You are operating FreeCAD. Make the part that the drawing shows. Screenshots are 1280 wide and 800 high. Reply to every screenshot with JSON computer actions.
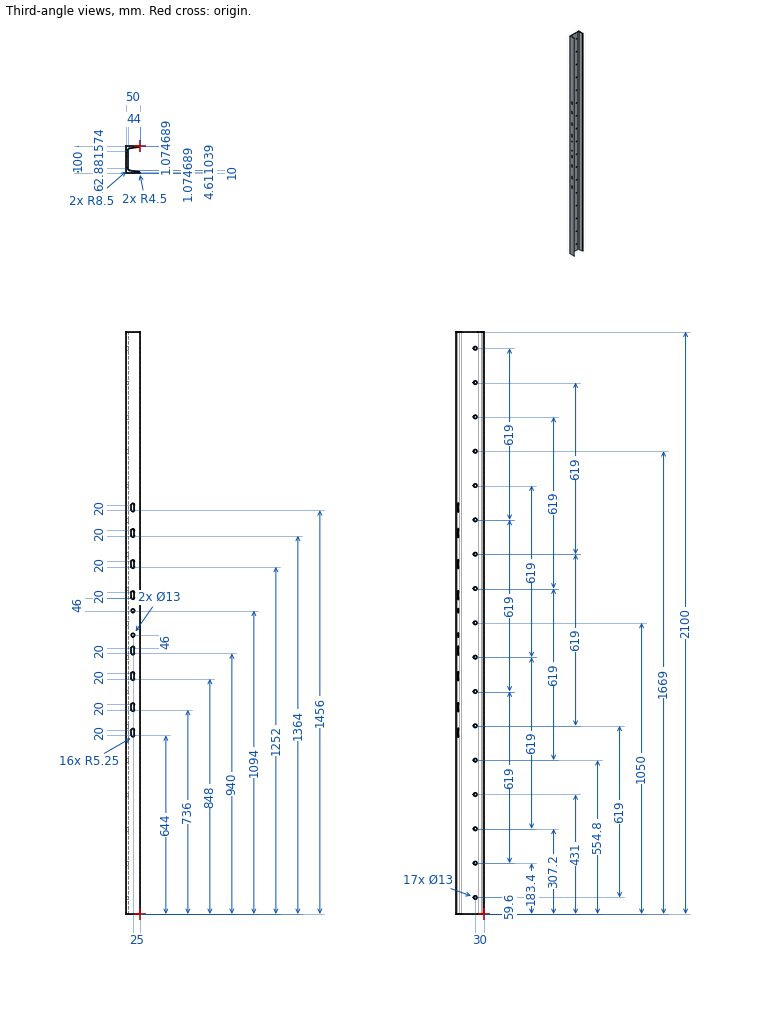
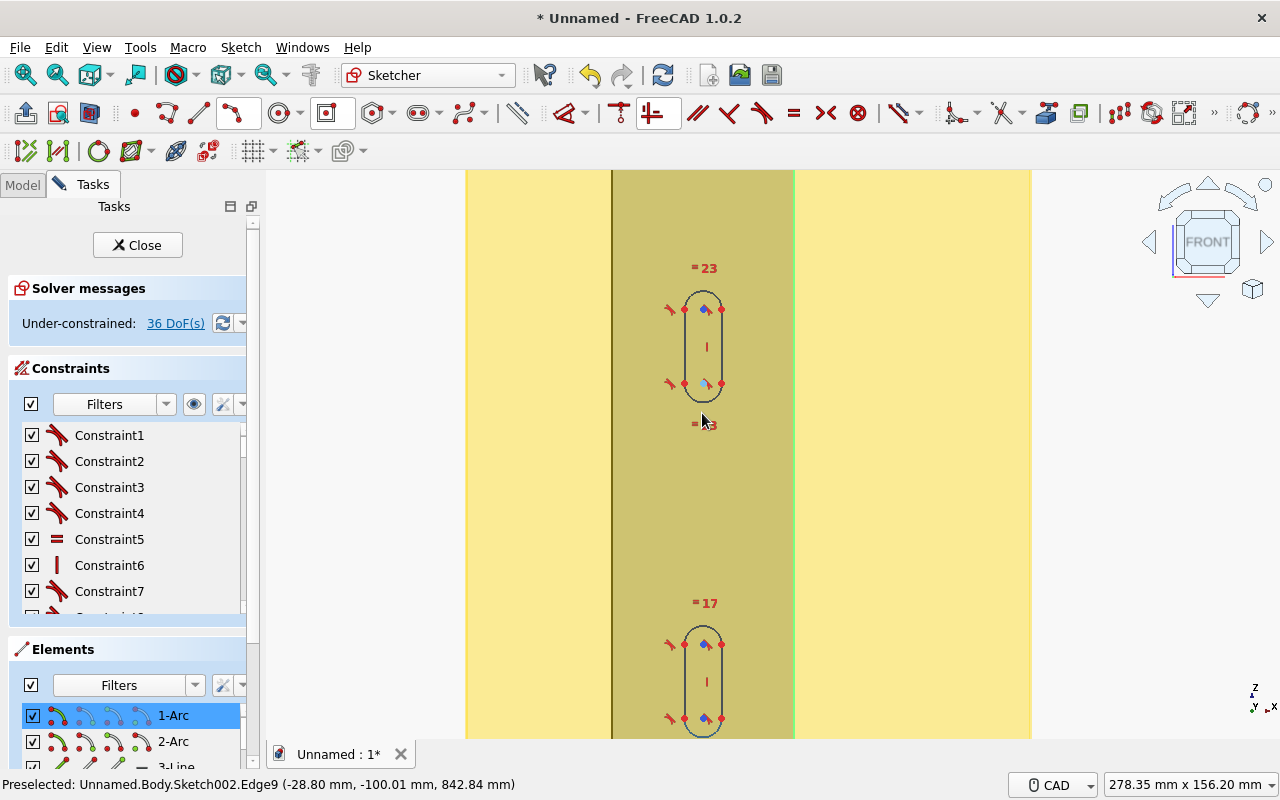
{"action": "left_click", "coordinate": [693, 399]}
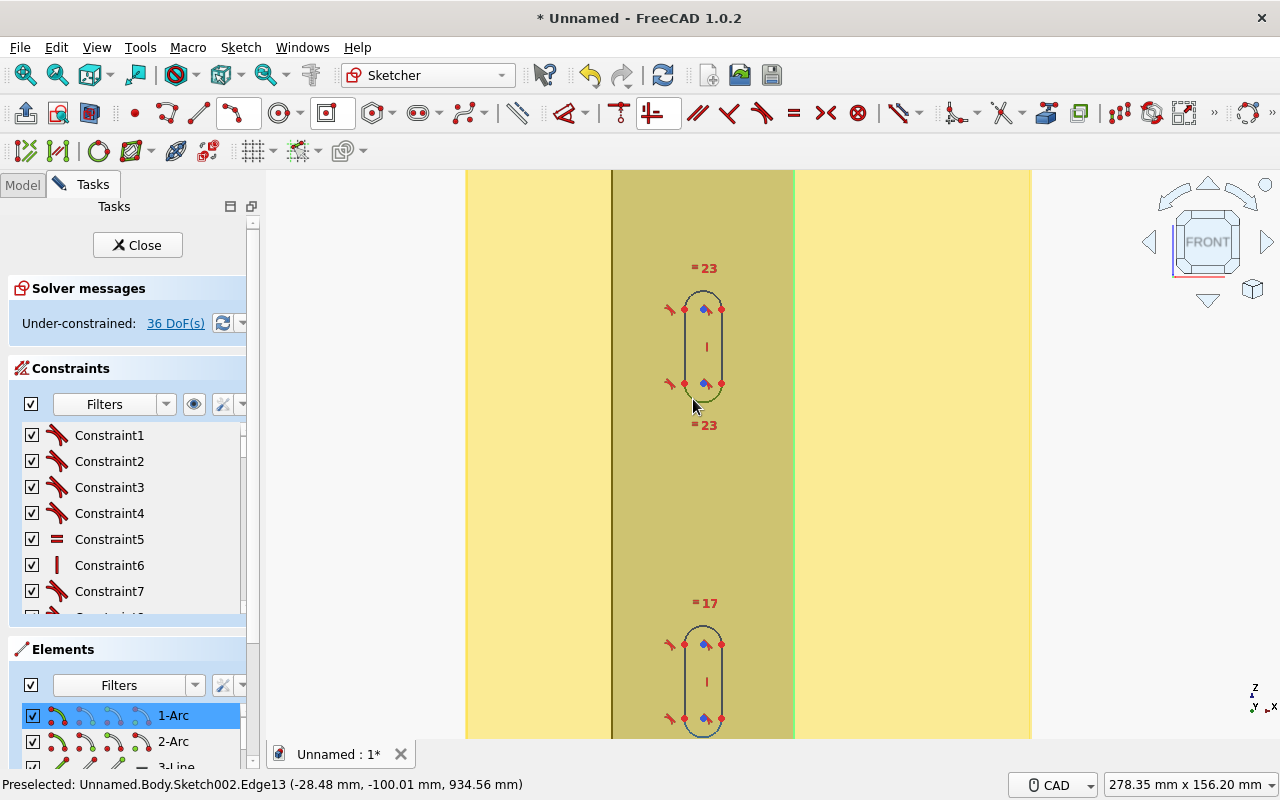
{"action": "scroll", "coordinate": [702, 413], "scroll_direction": "down", "scroll_amount": 14}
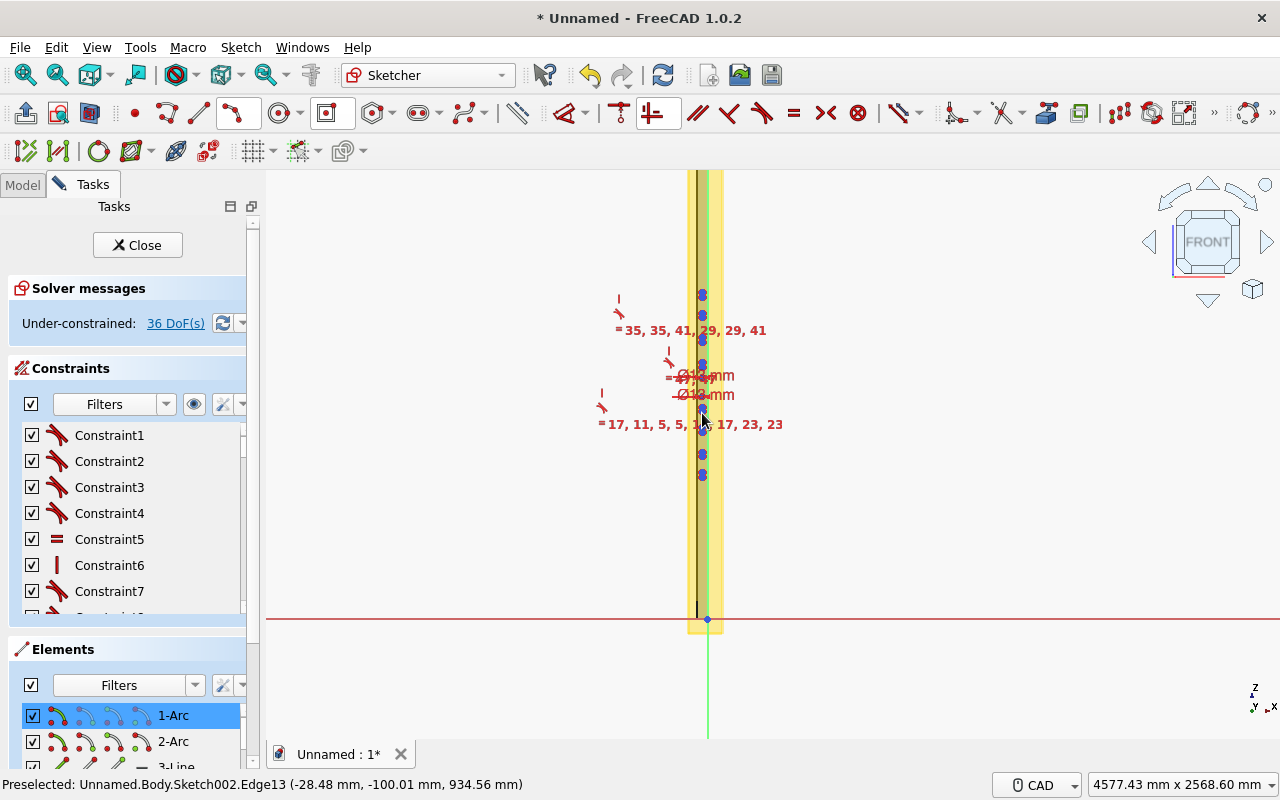
{"action": "scroll", "coordinate": [702, 343], "scroll_direction": "up", "scroll_amount": 14}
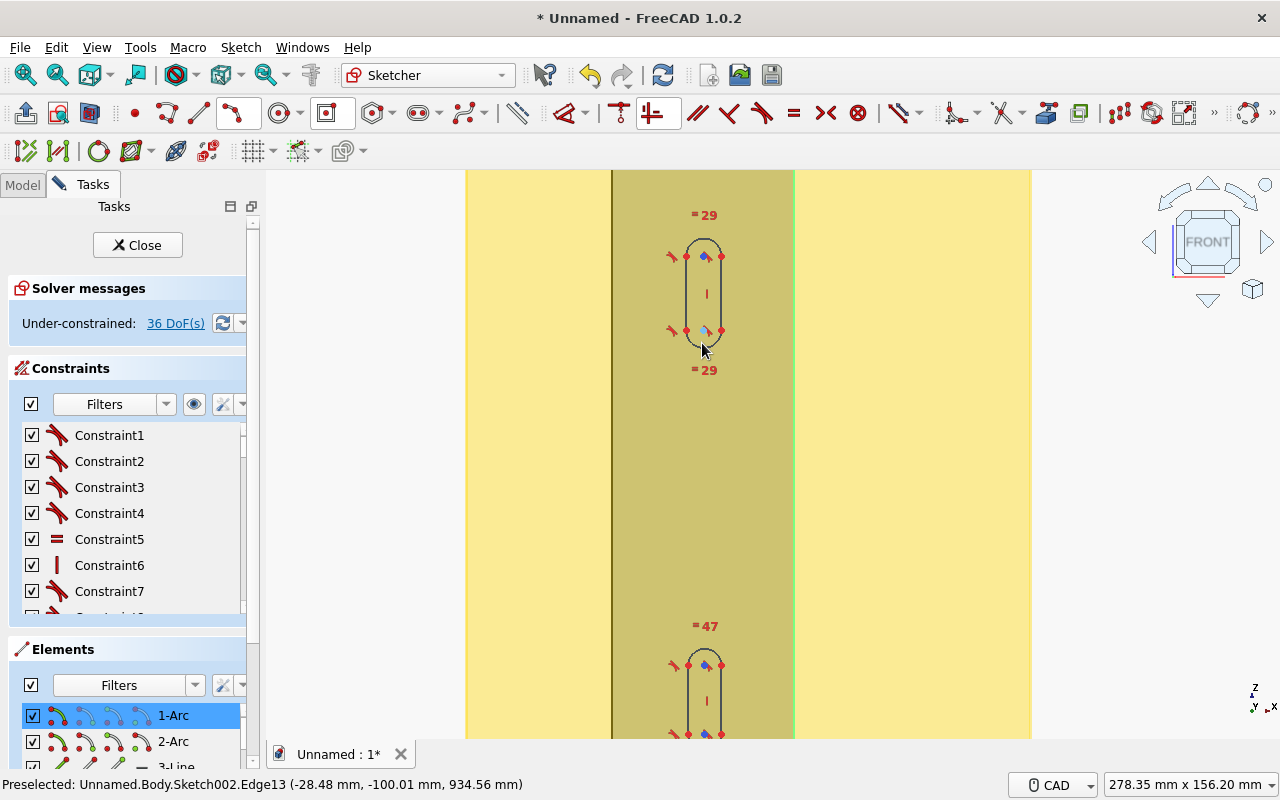
{"action": "left_click", "coordinate": [693, 345]}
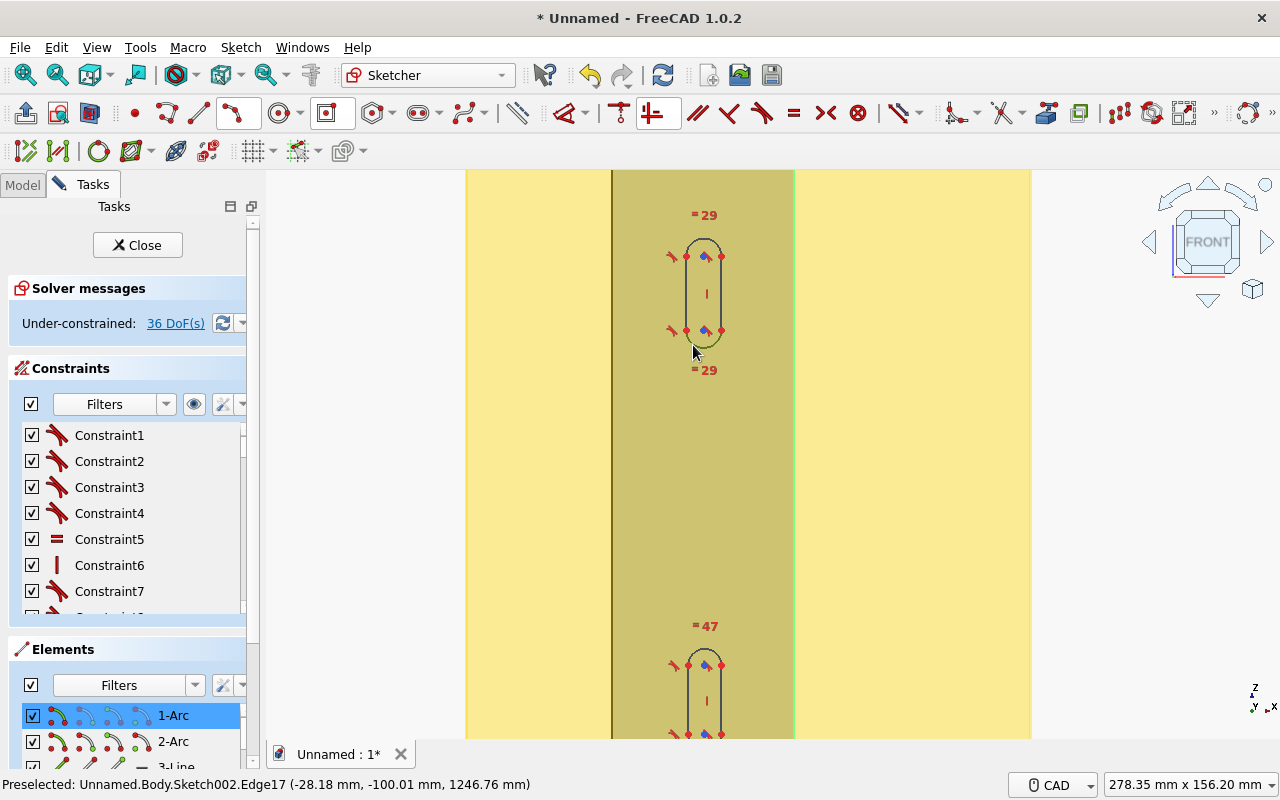
{"action": "scroll", "coordinate": [702, 342], "scroll_direction": "down", "scroll_amount": 14}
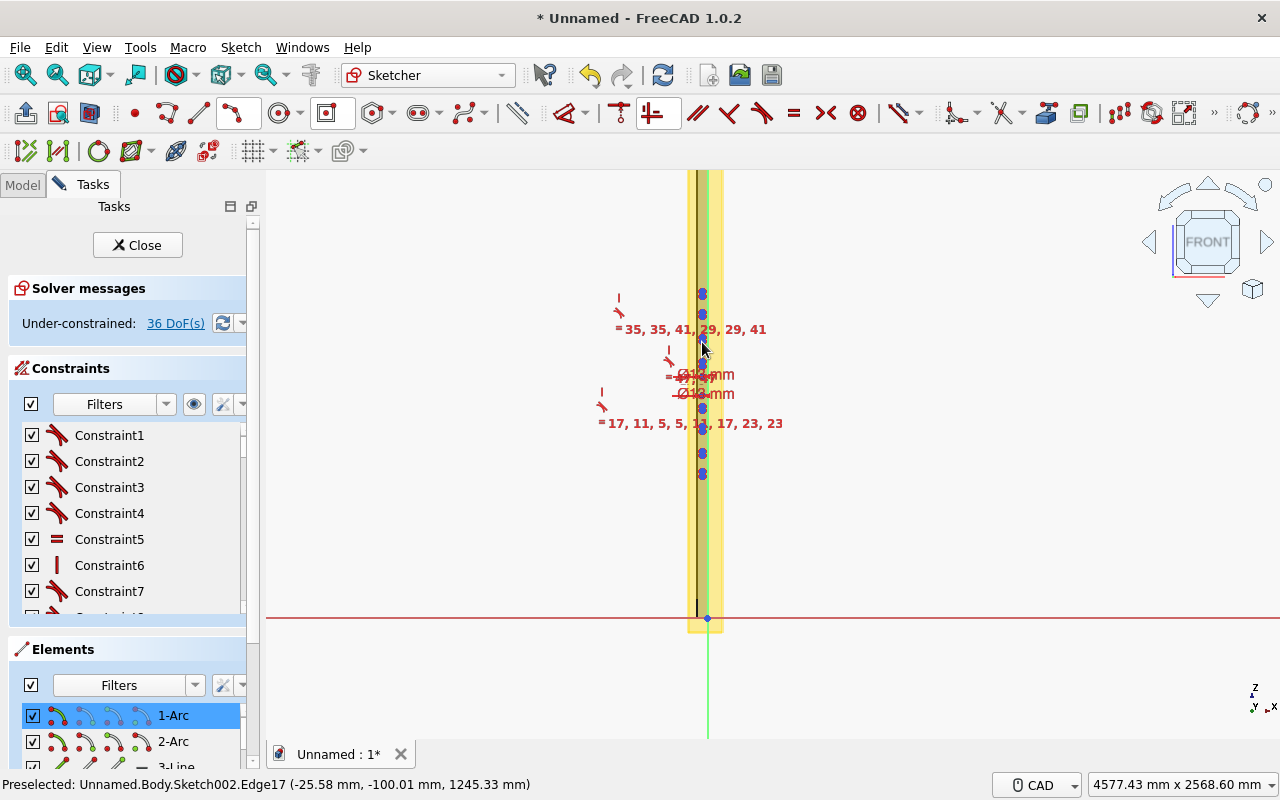
{"action": "scroll", "coordinate": [702, 297], "scroll_direction": "up", "scroll_amount": 14}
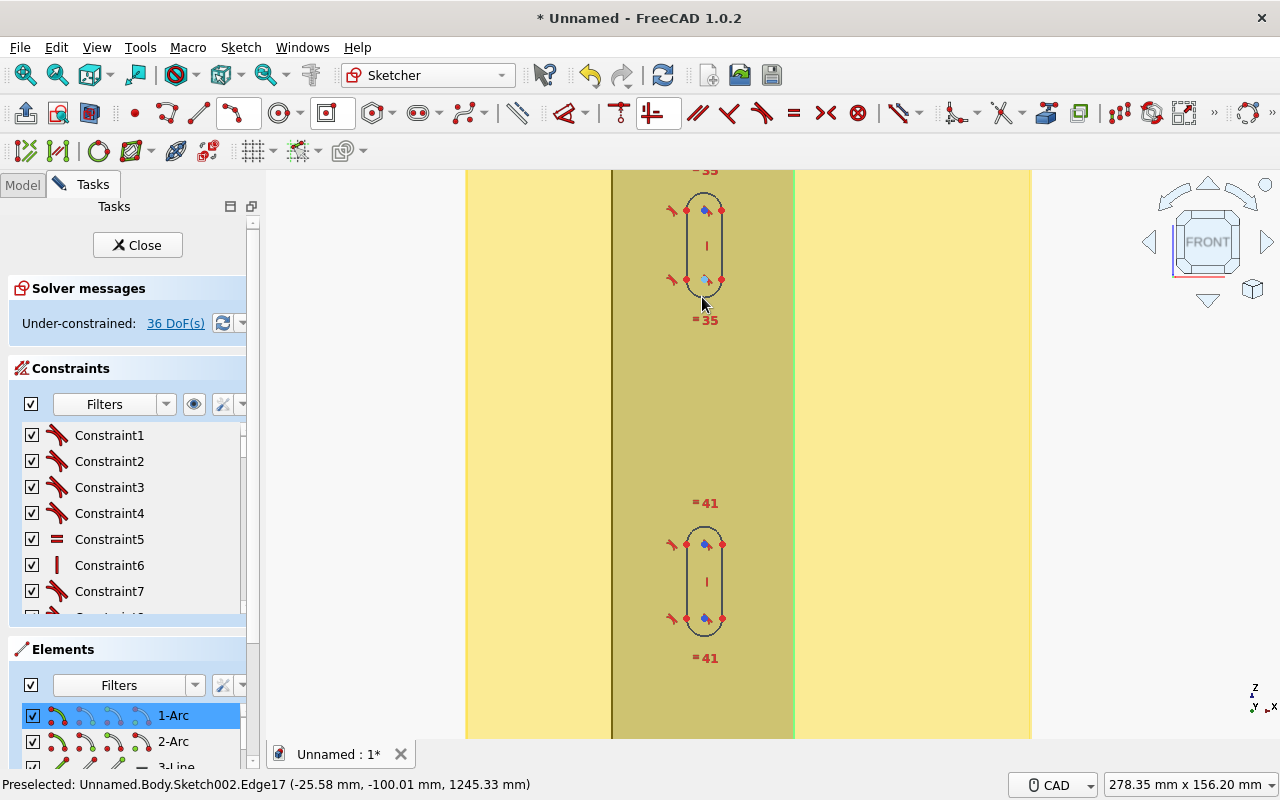
{"action": "left_click", "coordinate": [694, 294]}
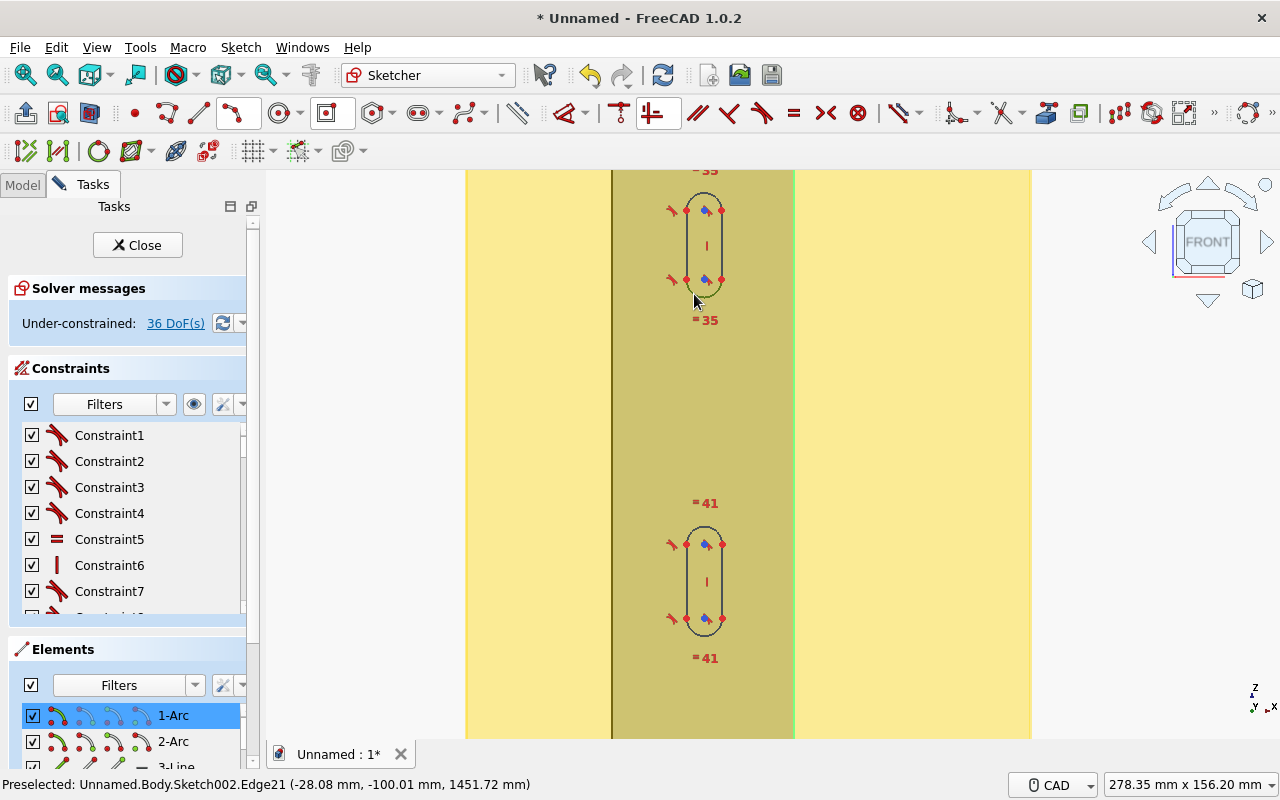
{"action": "left_click", "coordinate": [694, 633]}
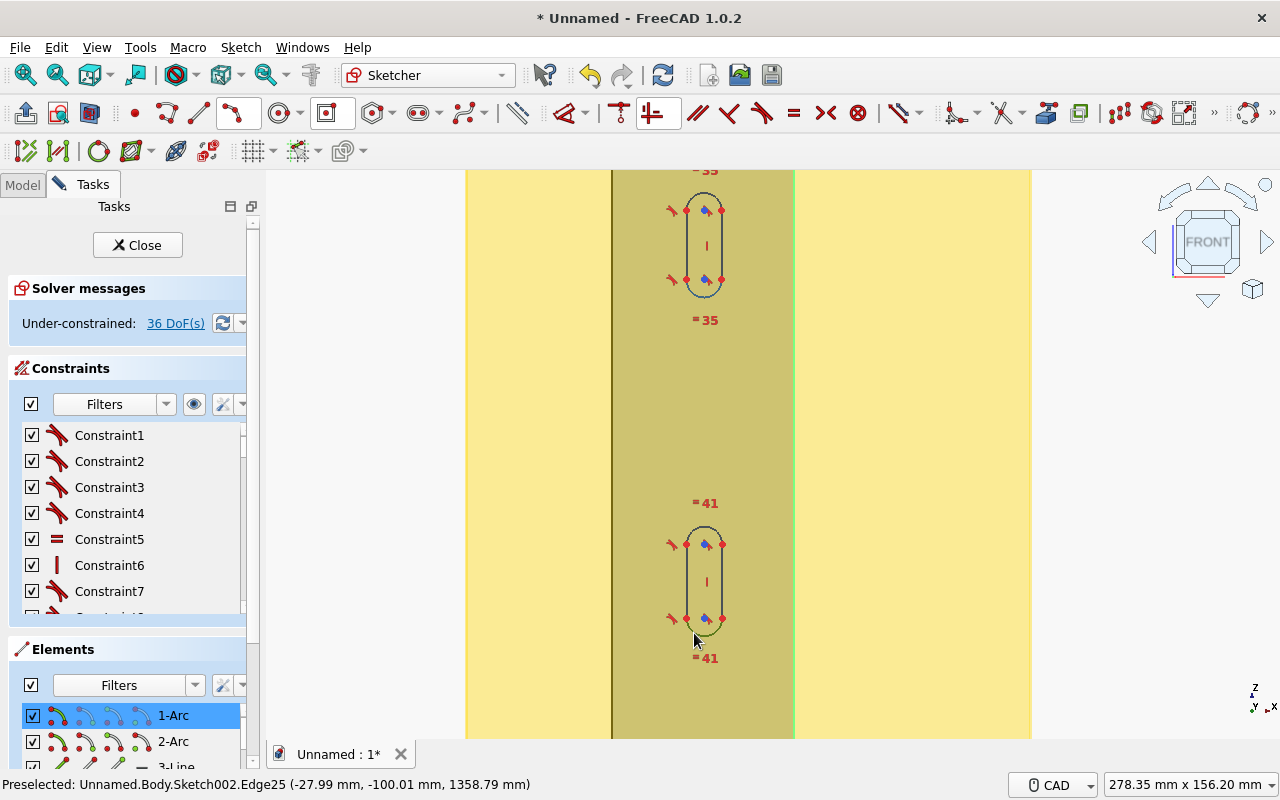
{"action": "scroll", "coordinate": [702, 297], "scroll_direction": "down", "scroll_amount": 14}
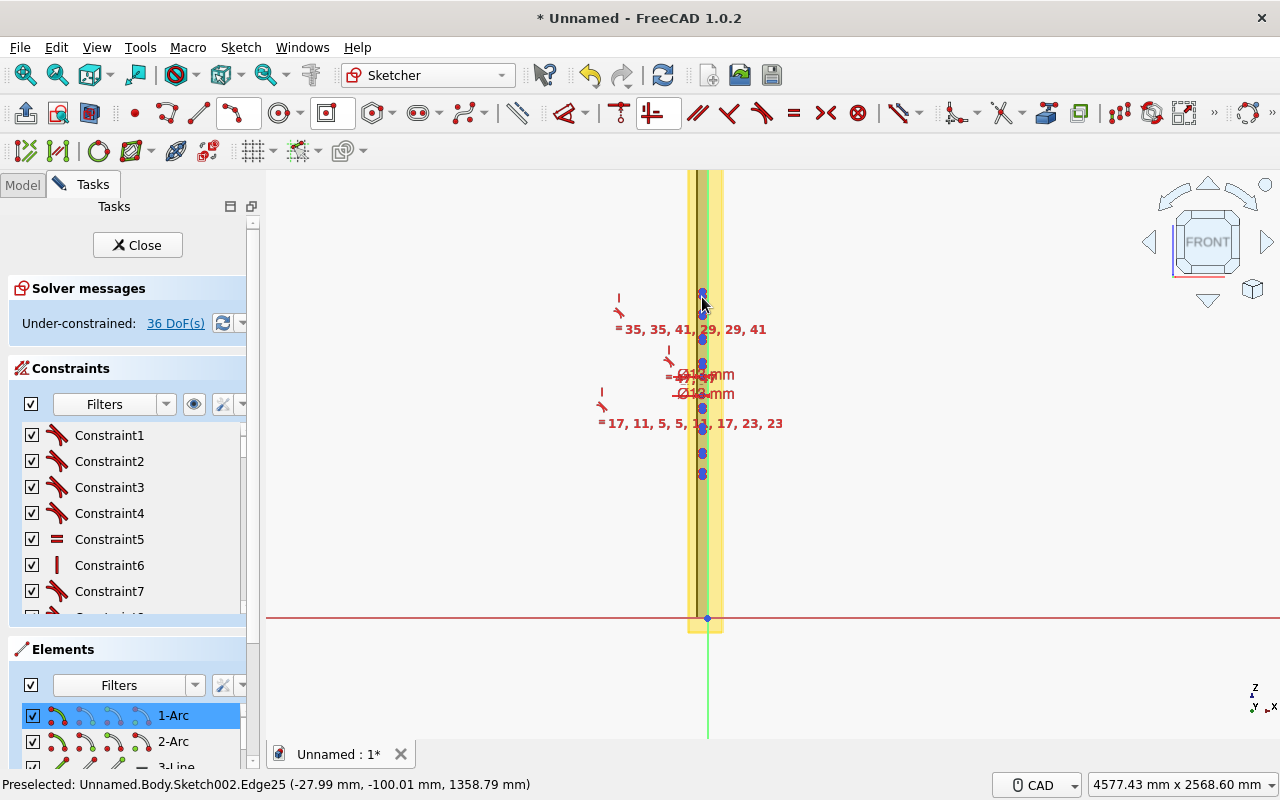
{"action": "scroll", "coordinate": [702, 367], "scroll_direction": "up", "scroll_amount": 14}